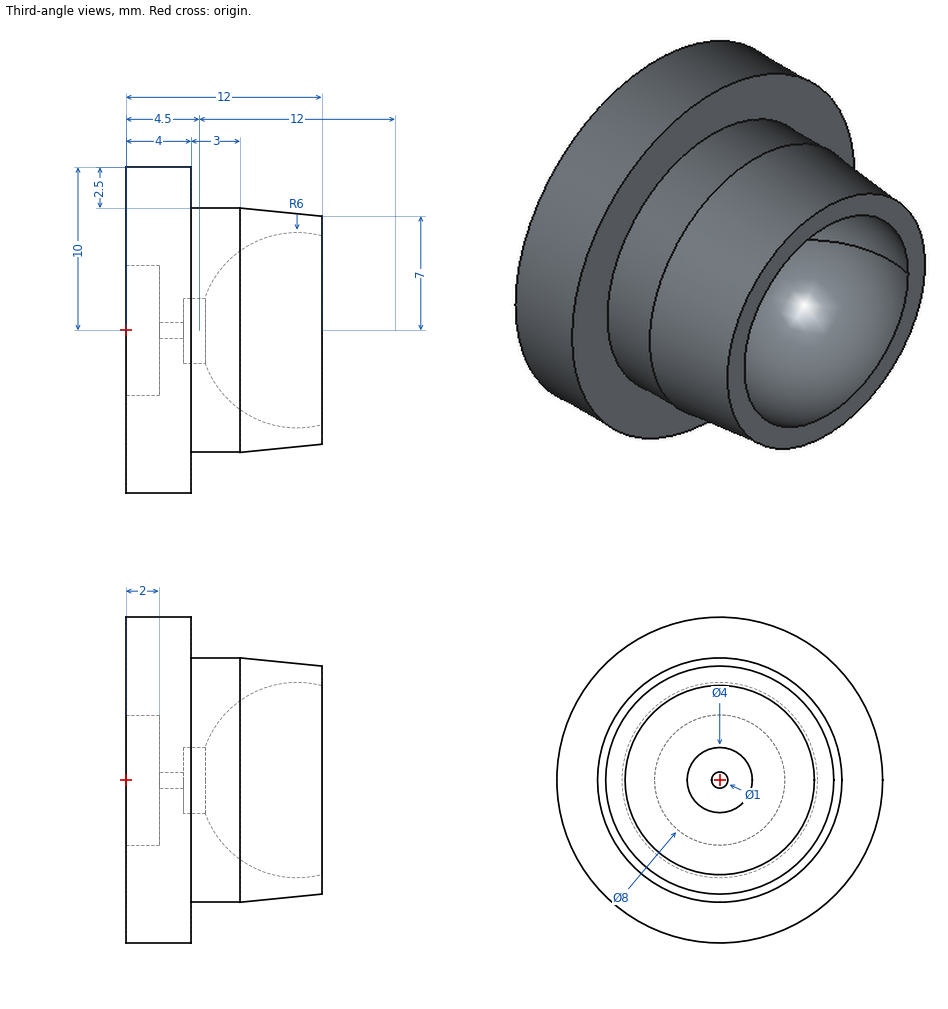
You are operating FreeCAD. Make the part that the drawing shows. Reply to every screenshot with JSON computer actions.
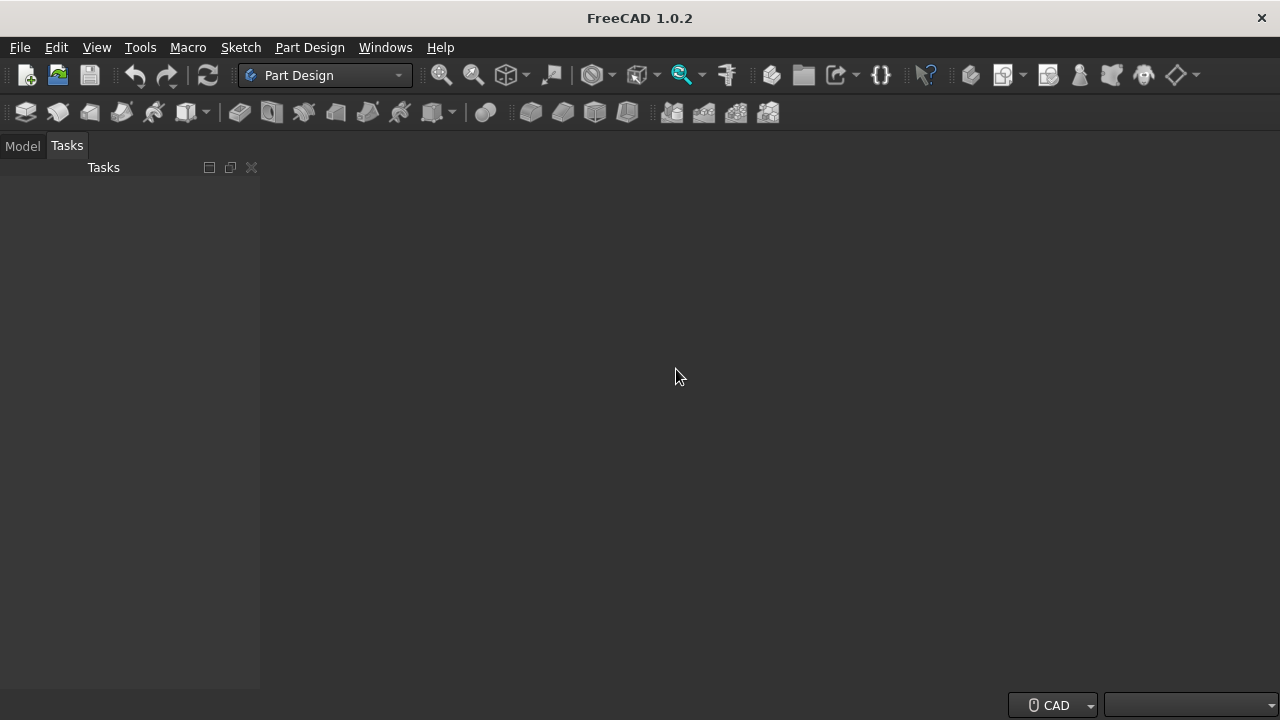
{"action": "left_click", "coordinate": [26, 76]}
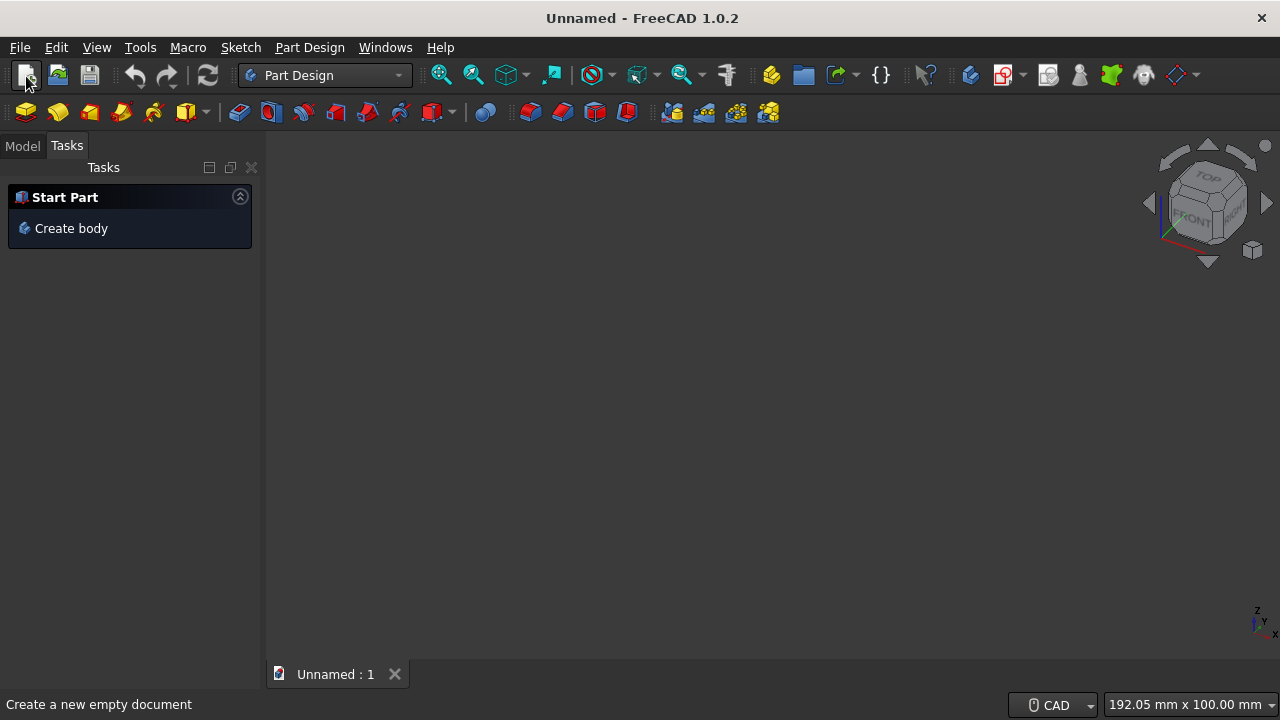
{"action": "left_click", "coordinate": [1004, 76]}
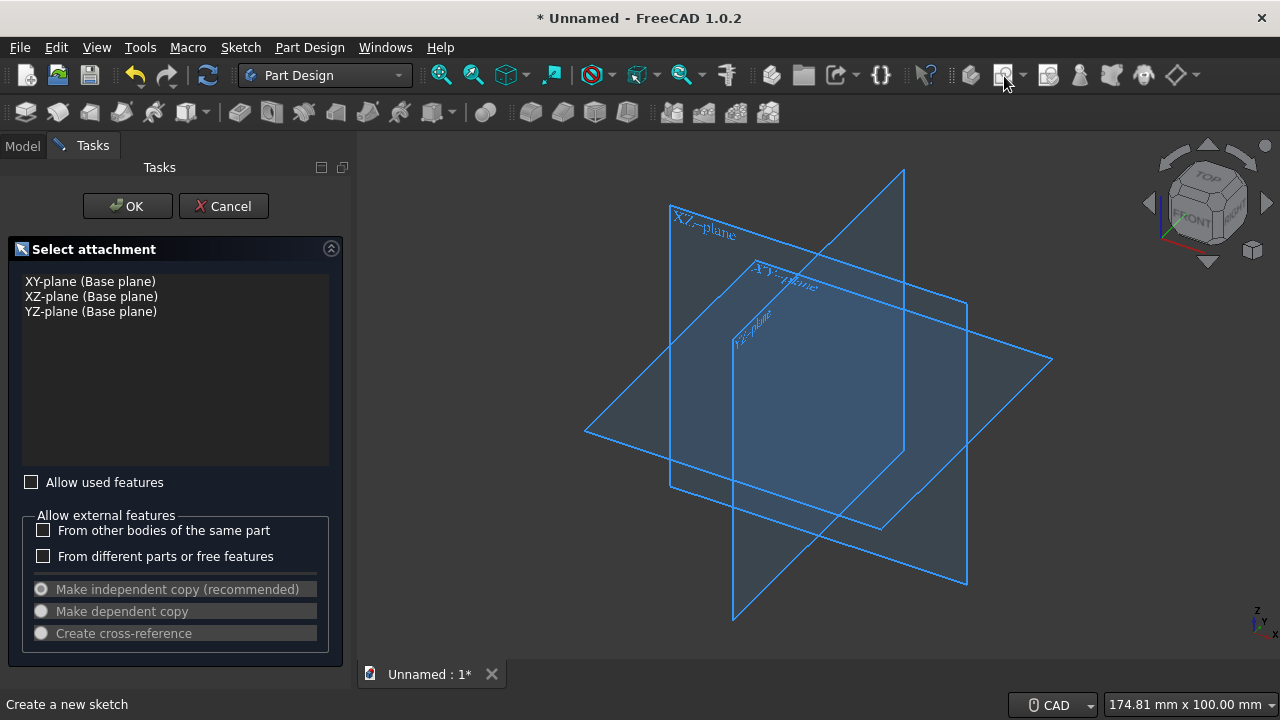
{"action": "left_click", "coordinate": [82, 282]}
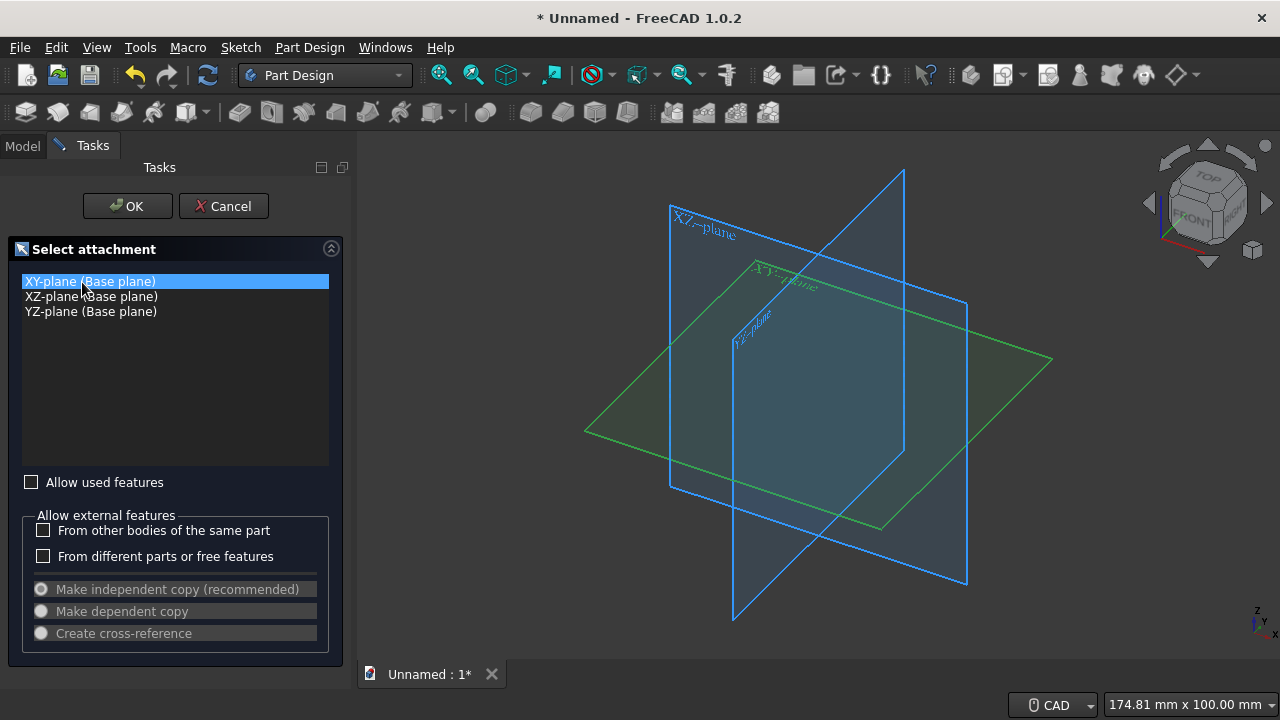
{"action": "left_click", "coordinate": [128, 206]}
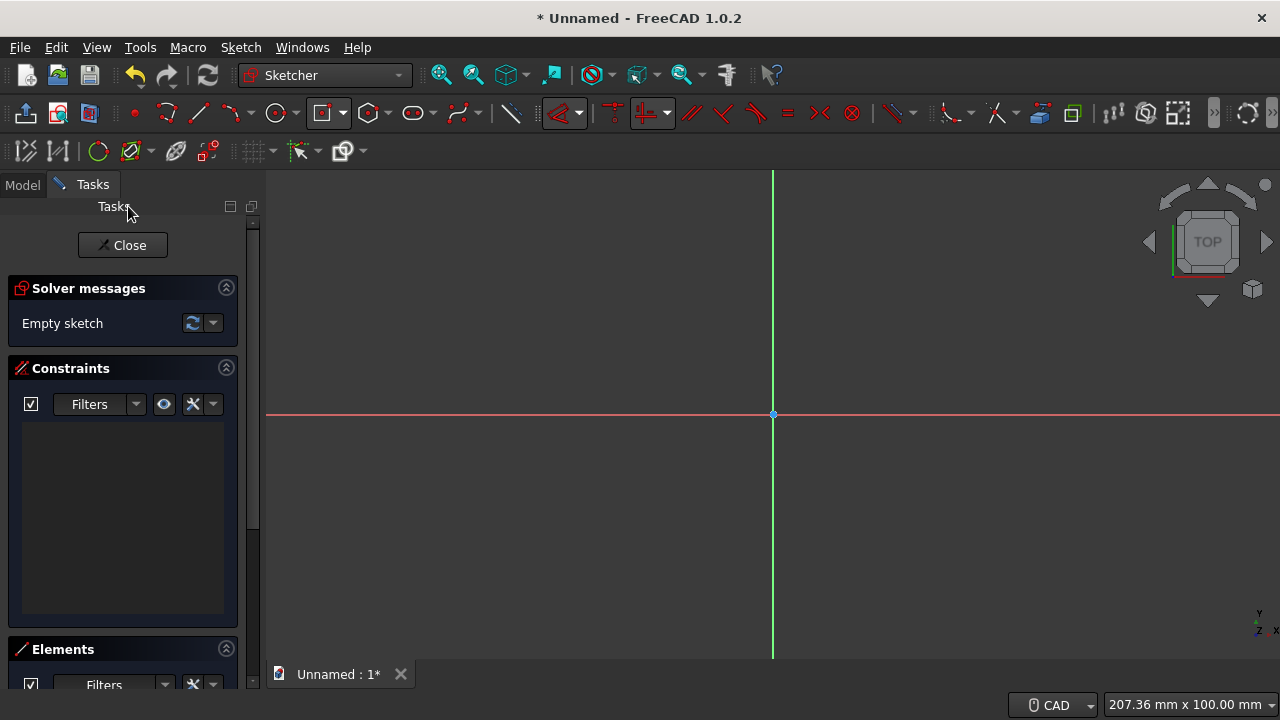
{"action": "scroll", "coordinate": [822, 385], "scroll_direction": "up", "scroll_amount": 9}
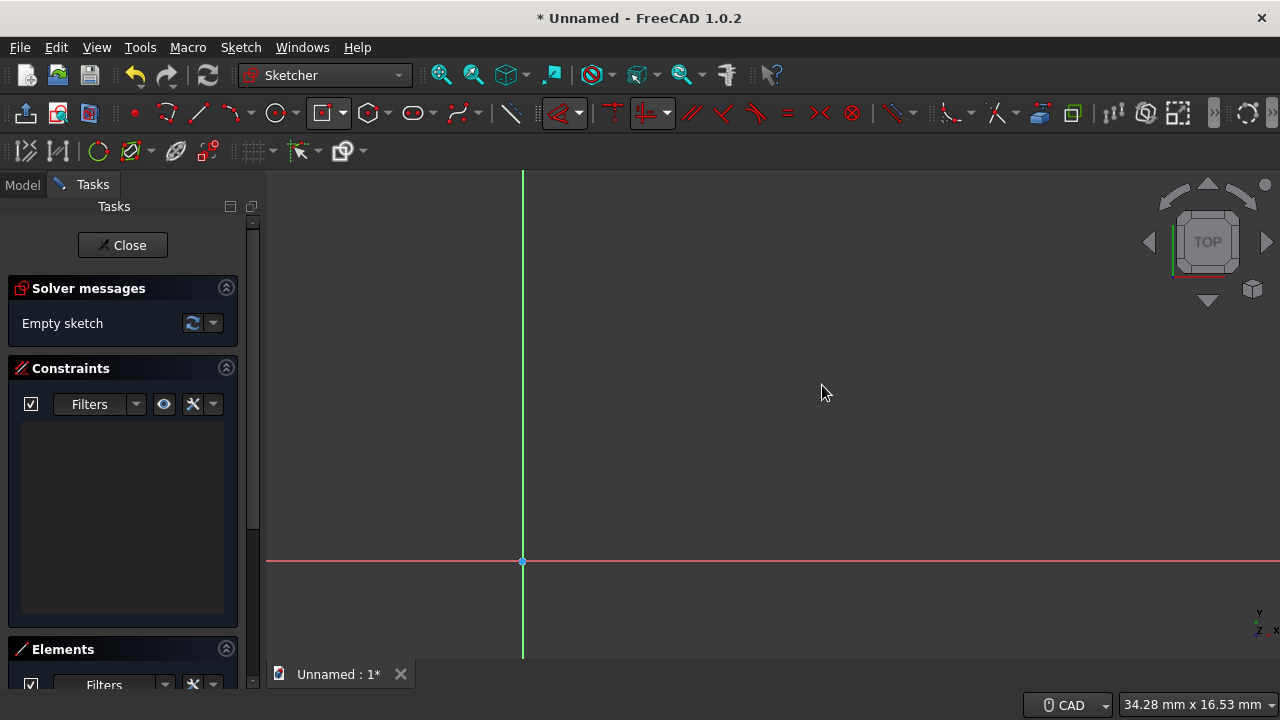
{"action": "left_click", "coordinate": [168, 114]}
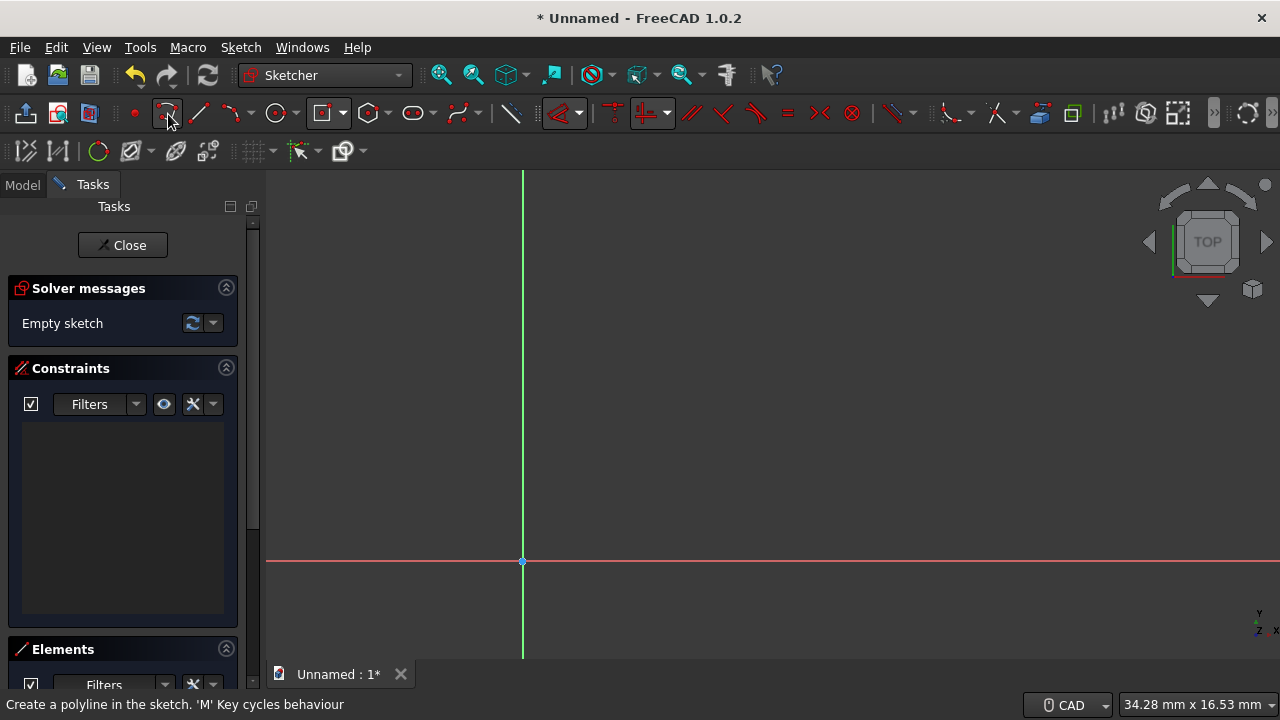
{"action": "left_click", "coordinate": [523, 561]}
{"action": "left_click", "coordinate": [878, 552]}
{"action": "left_click", "coordinate": [878, 354]}
{"action": "left_click", "coordinate": [730, 339]}
{"action": "left_click", "coordinate": [641, 339]}
{"action": "left_click", "coordinate": [641, 265]}
{"action": "left_click", "coordinate": [532, 265]}
{"action": "left_click", "coordinate": [523, 561]}
{"action": "key", "text": "Escape"}
{"action": "key", "text": "Escape"}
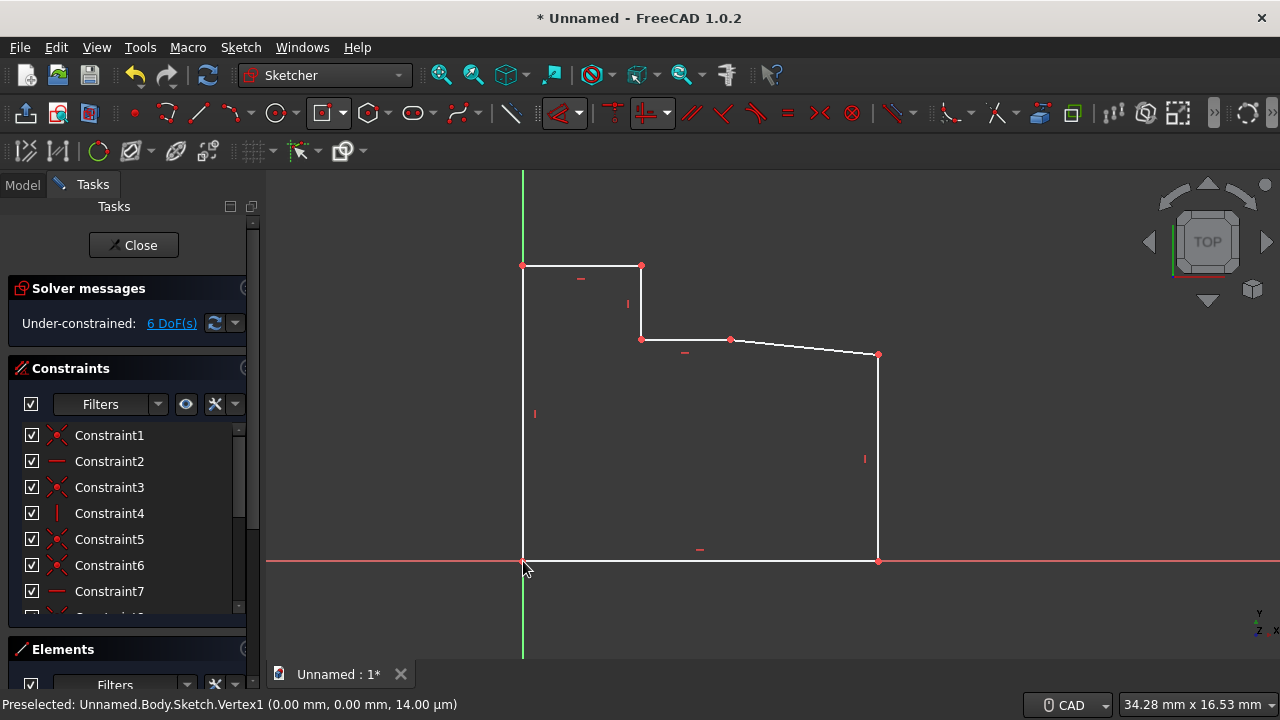
{"action": "left_click", "coordinate": [558, 114]}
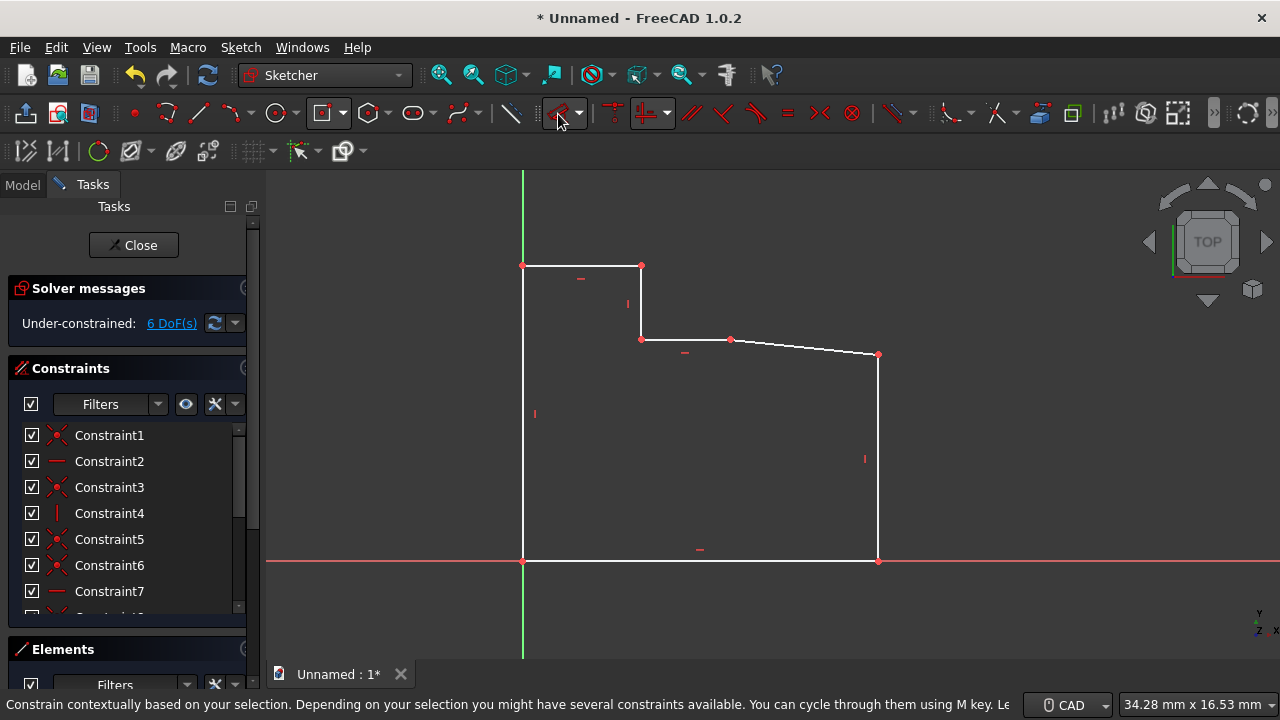
{"action": "left_click", "coordinate": [878, 499]}
{"action": "left_click", "coordinate": [912, 458]}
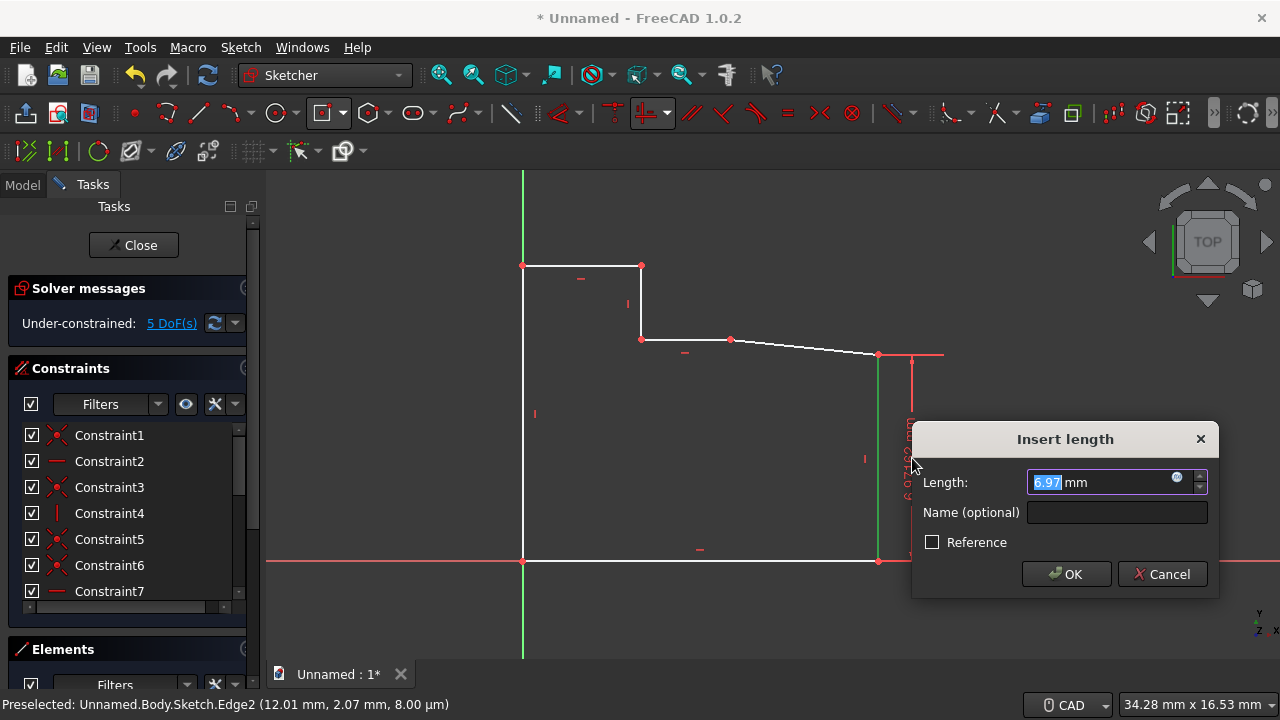
{"action": "type", "text": "7"}
{"action": "key", "text": "Return"}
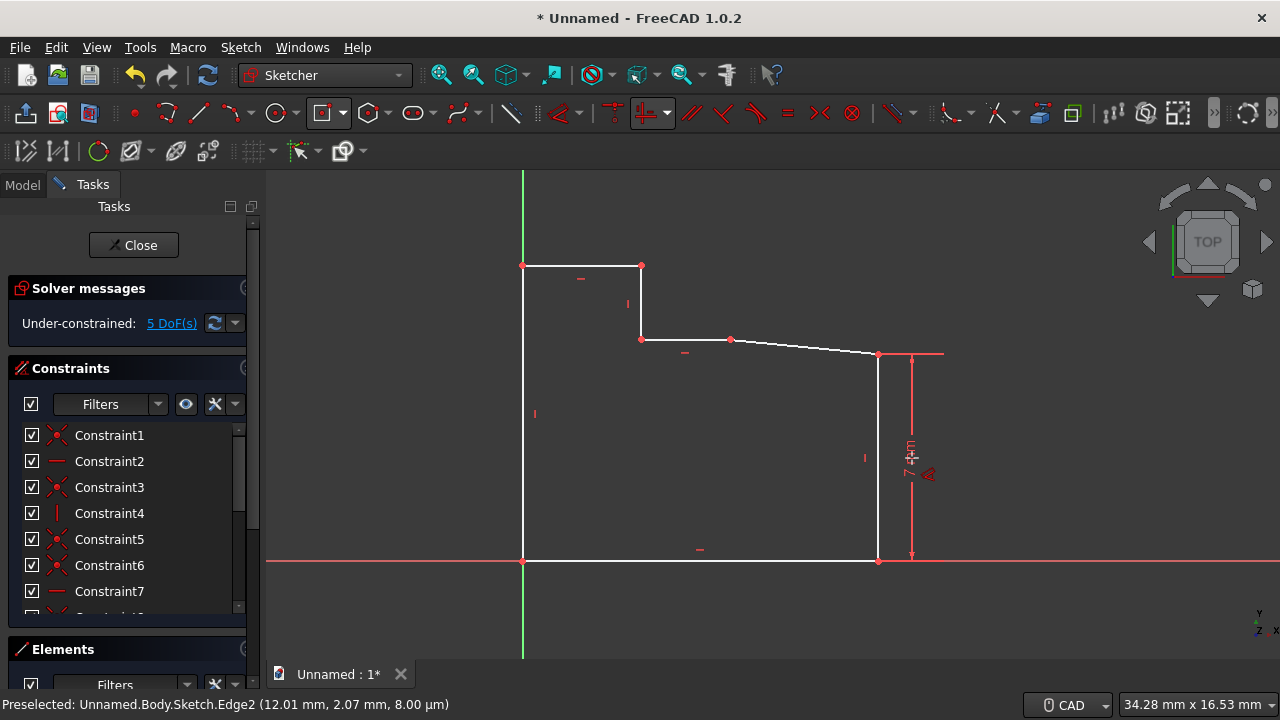
{"action": "left_click", "coordinate": [703, 340]}
{"action": "left_click", "coordinate": [685, 306]}